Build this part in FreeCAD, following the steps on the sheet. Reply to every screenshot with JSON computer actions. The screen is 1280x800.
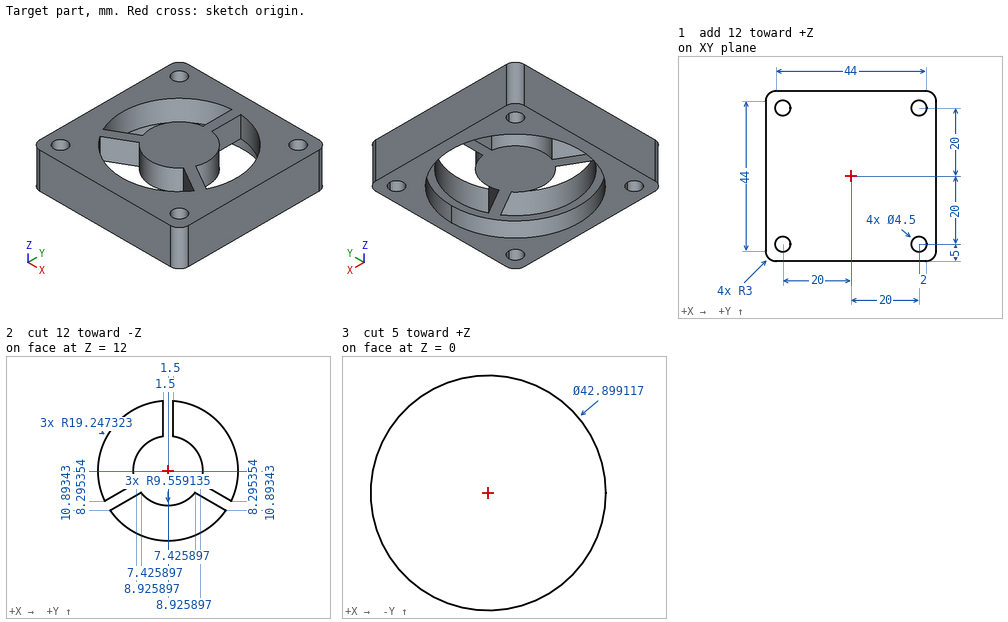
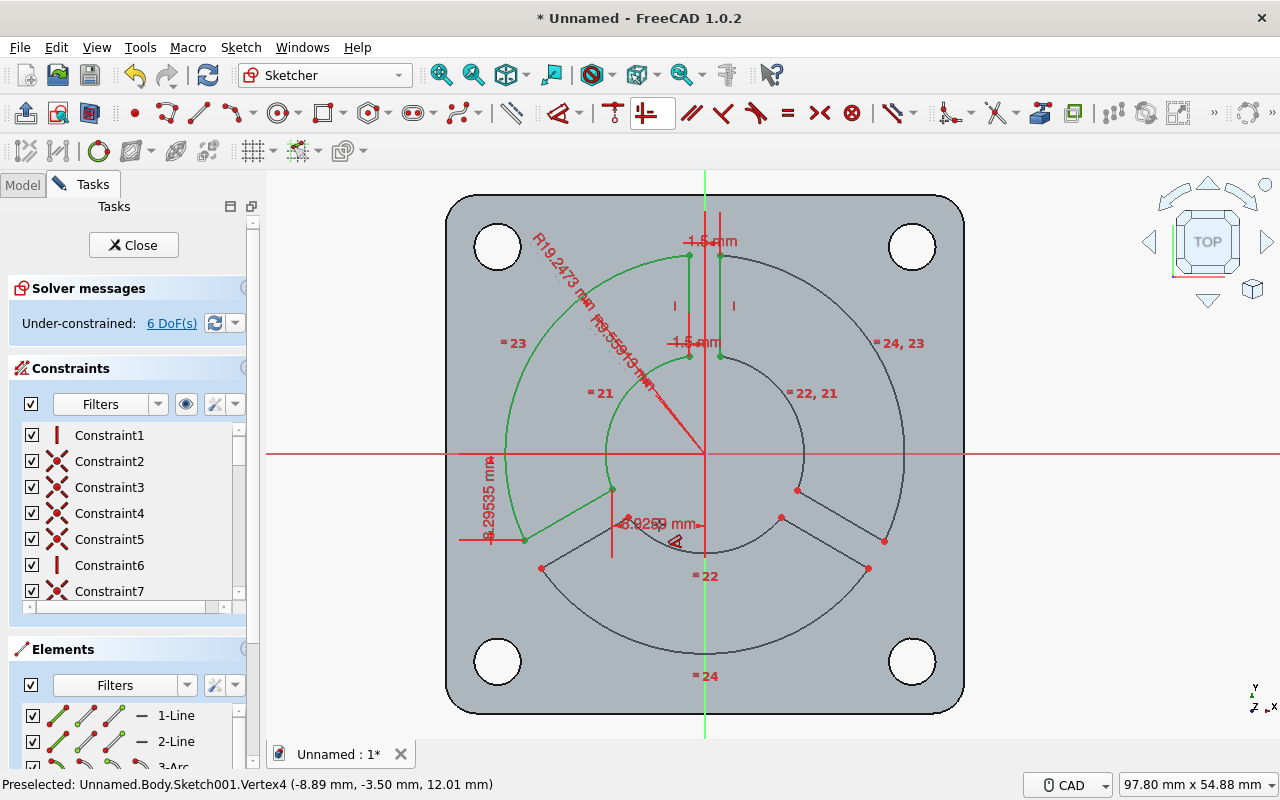
{"action": "left_click", "coordinate": [797, 491]}
{"action": "left_click", "coordinate": [751, 525]}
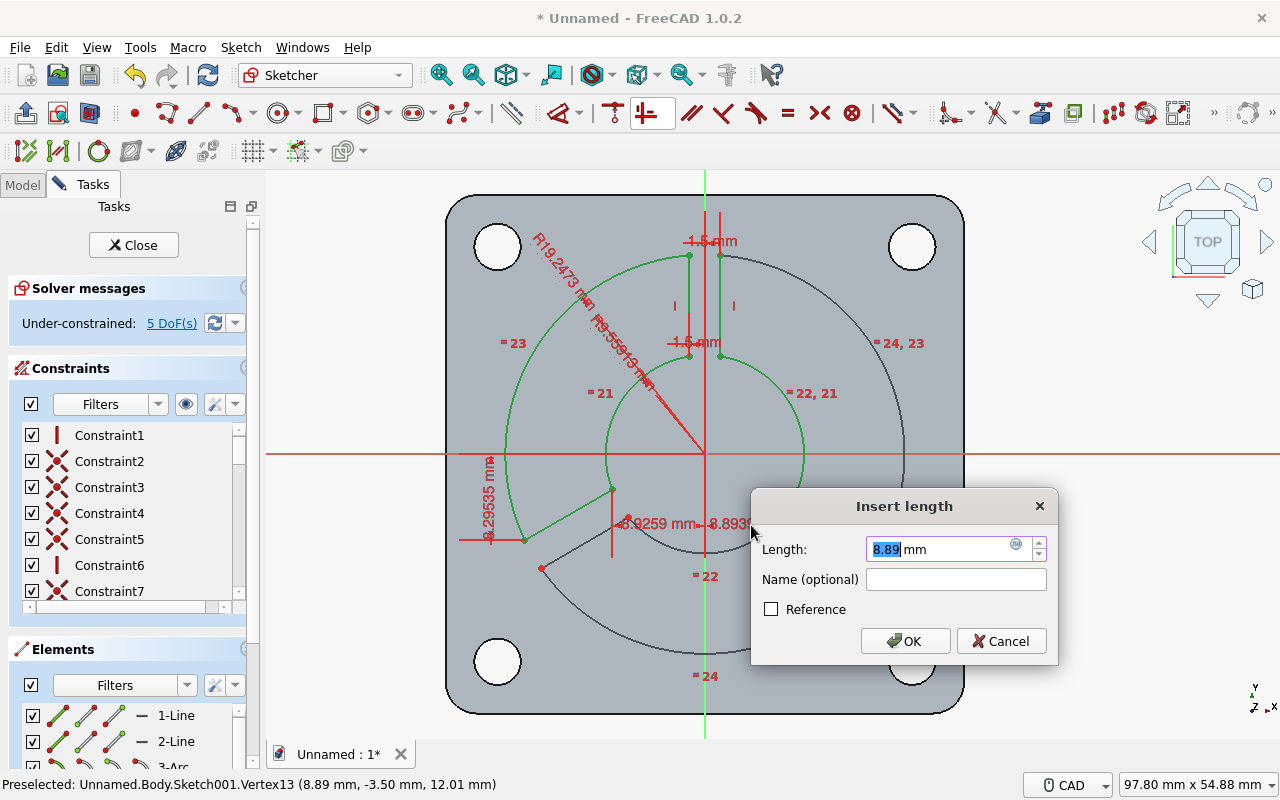
{"action": "type", "text": "8.925897"}
{"action": "key", "text": "Return"}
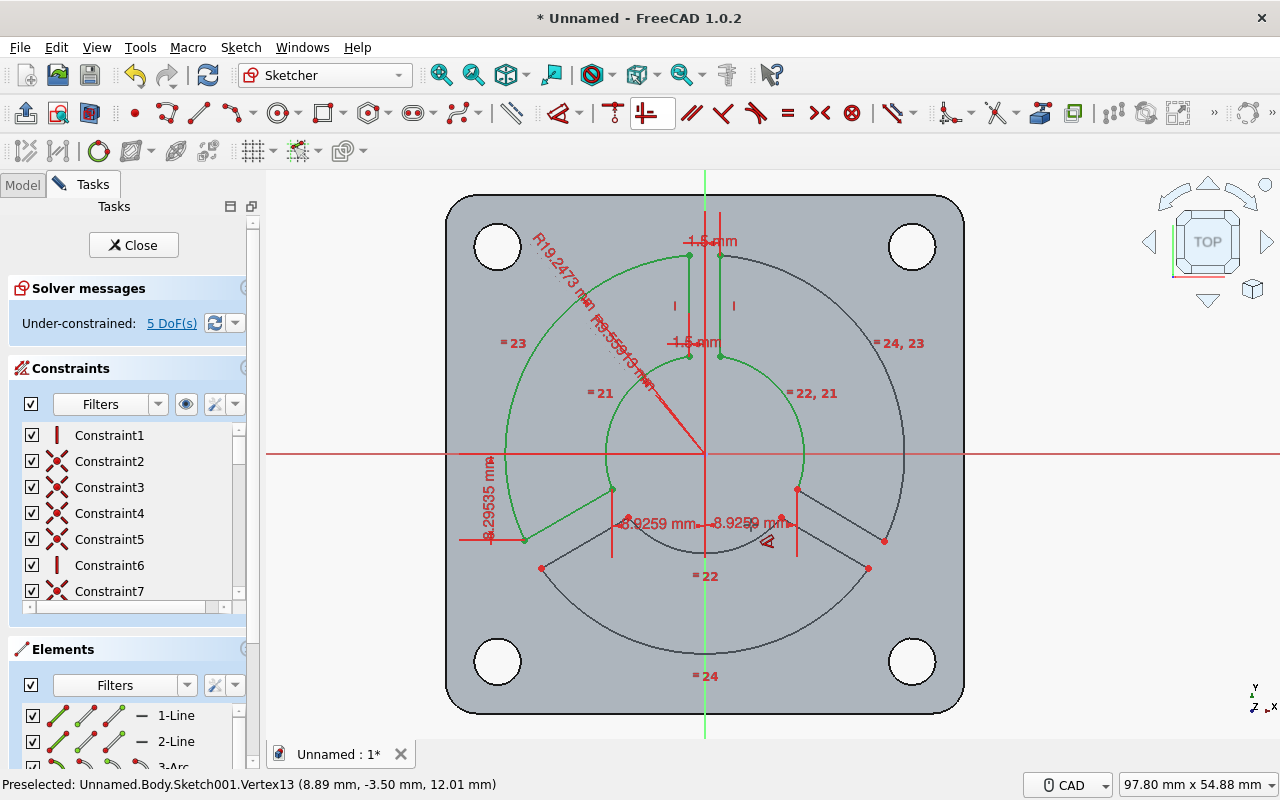
{"action": "left_click", "coordinate": [884, 542]}
{"action": "left_click", "coordinate": [918, 498]}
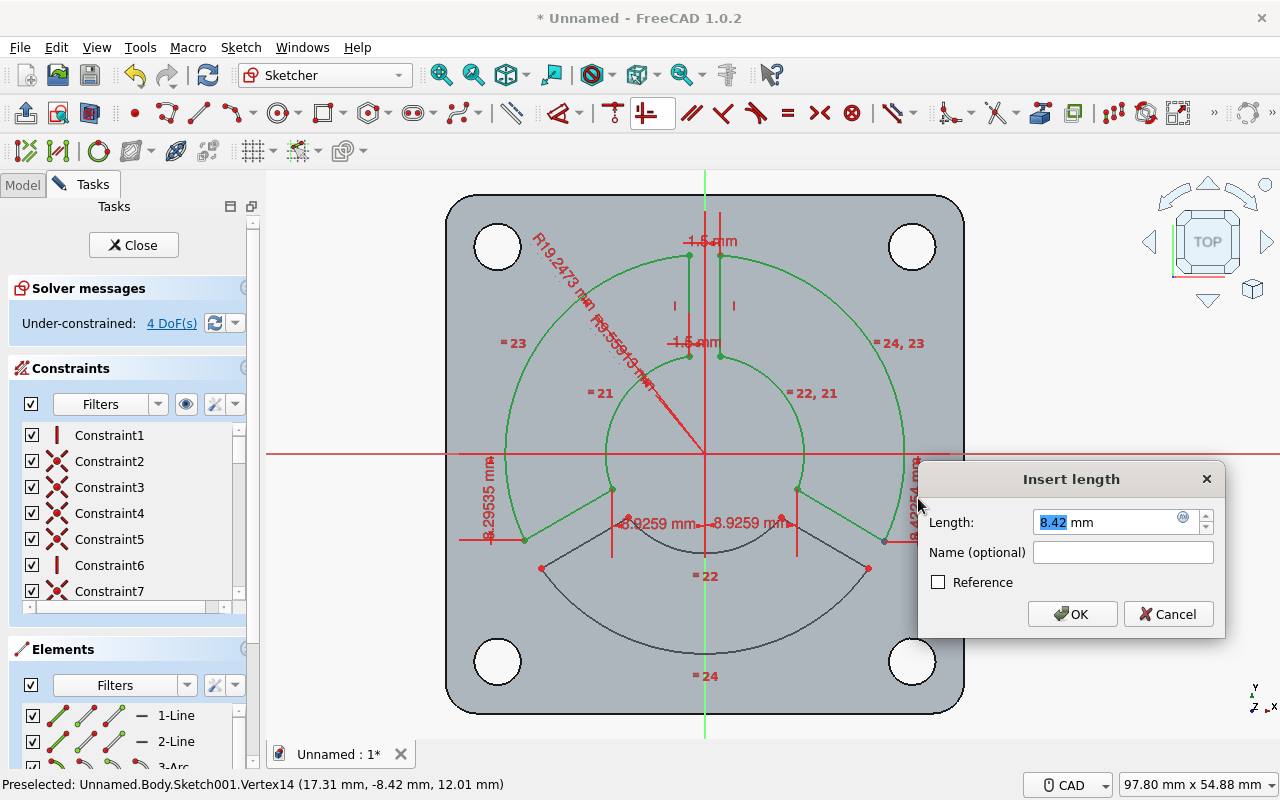
{"action": "type", "text": "8.295354"}
{"action": "key", "text": "Return"}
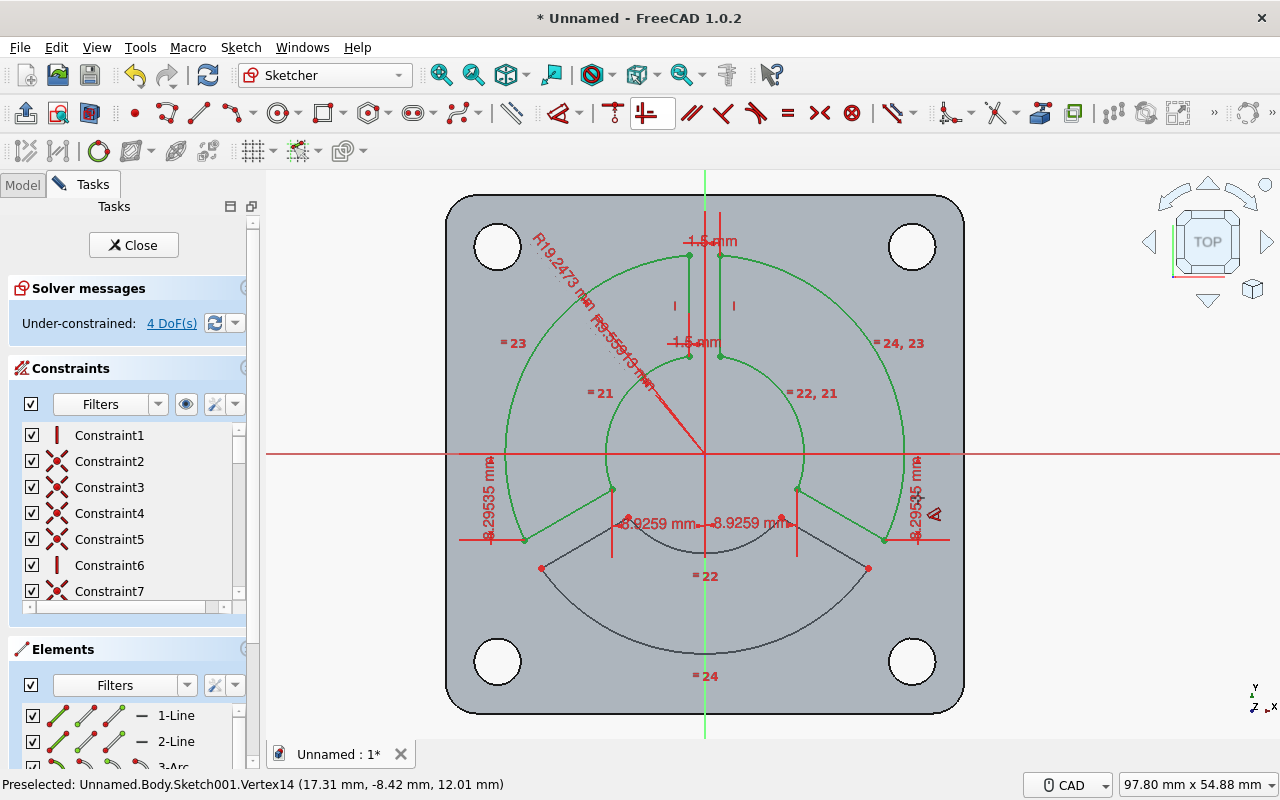
{"action": "left_click", "coordinate": [868, 569]}
{"action": "left_click", "coordinate": [902, 538]}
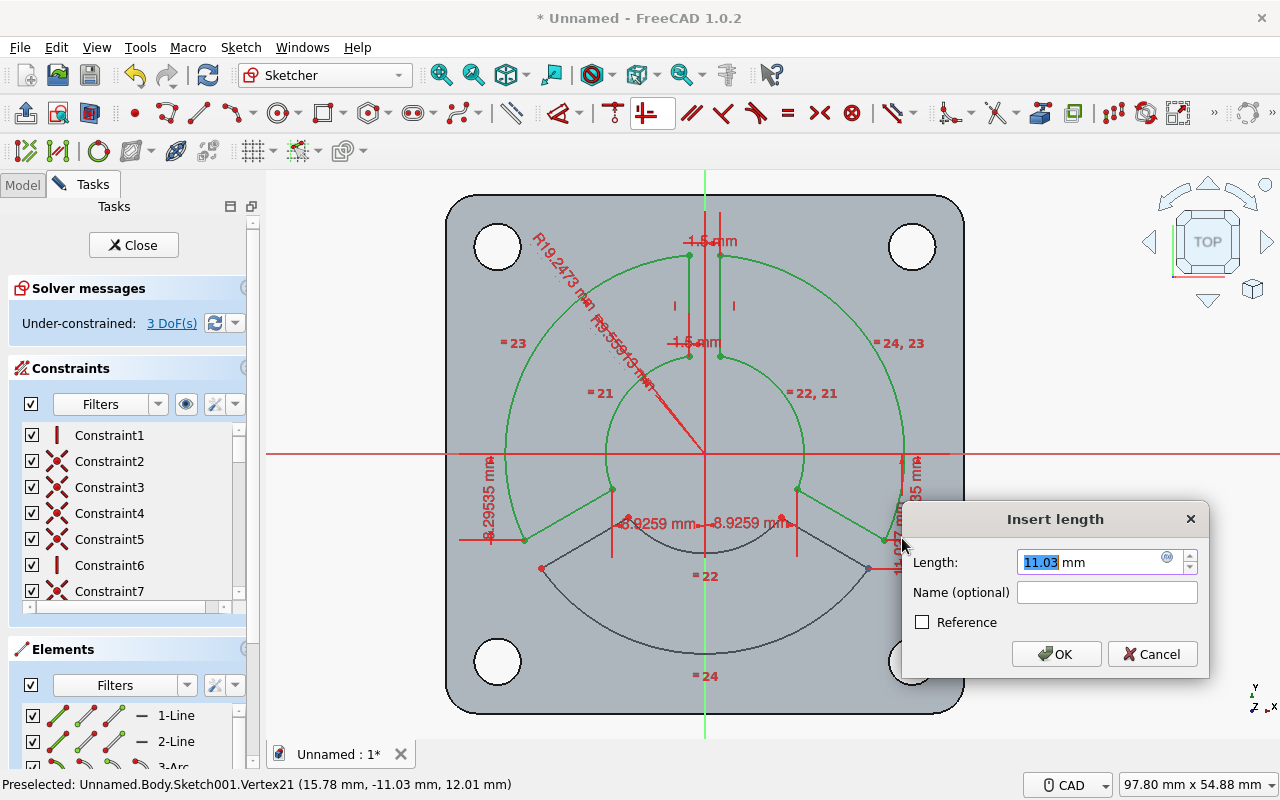
{"action": "type", "text": "10.89343"}
{"action": "key", "text": "Return"}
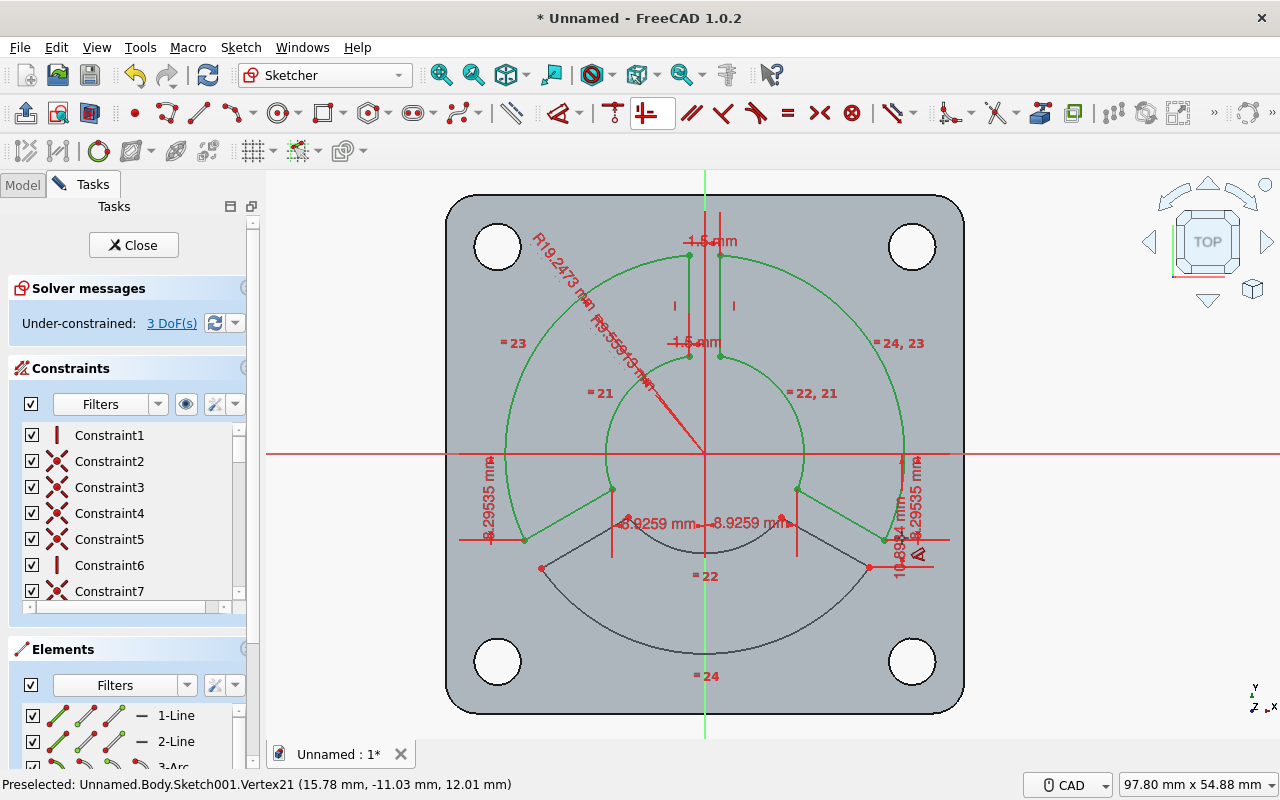
{"action": "left_click", "coordinate": [781, 518]}
{"action": "left_click", "coordinate": [761, 552]}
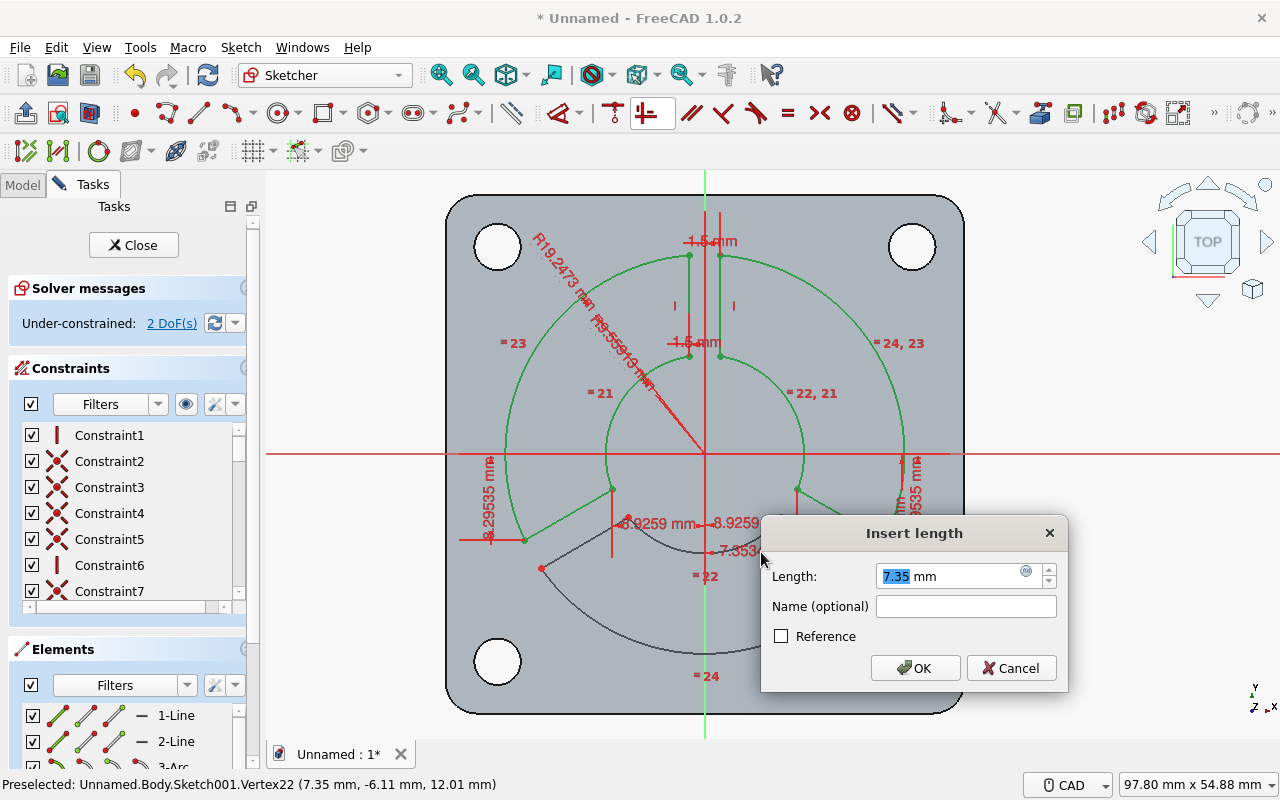
{"action": "type", "text": "7.425897"}
{"action": "key", "text": "Return"}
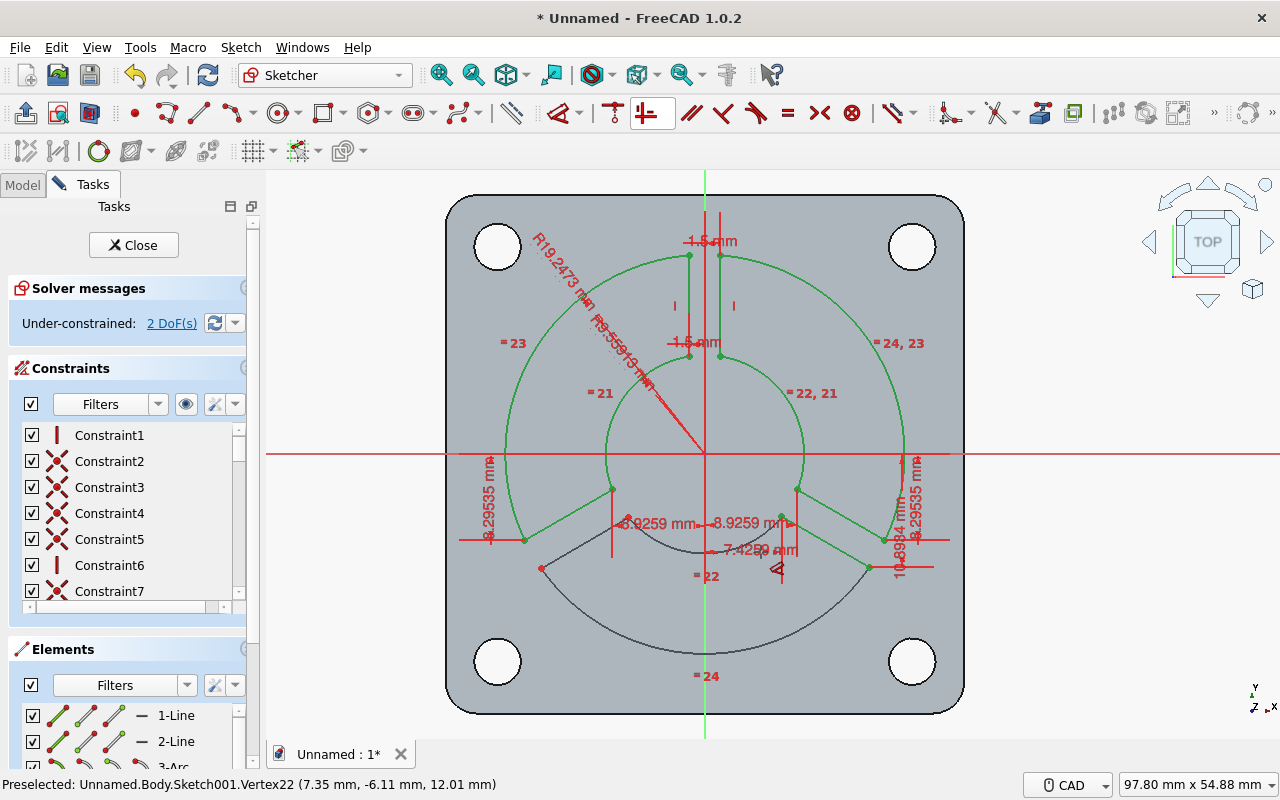
{"action": "left_click", "coordinate": [629, 518]}
{"action": "left_click", "coordinate": [649, 552]}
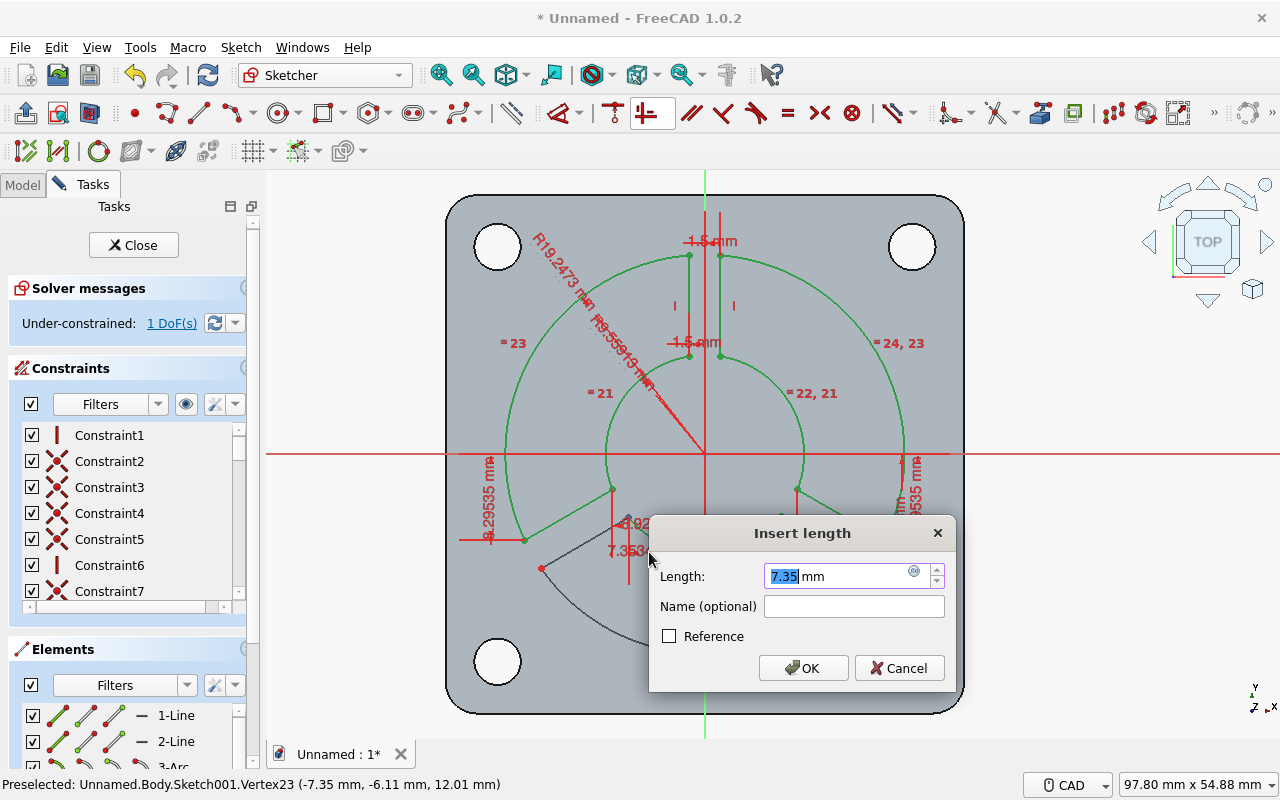
{"action": "type", "text": "7.425897"}
{"action": "key", "text": "Return"}